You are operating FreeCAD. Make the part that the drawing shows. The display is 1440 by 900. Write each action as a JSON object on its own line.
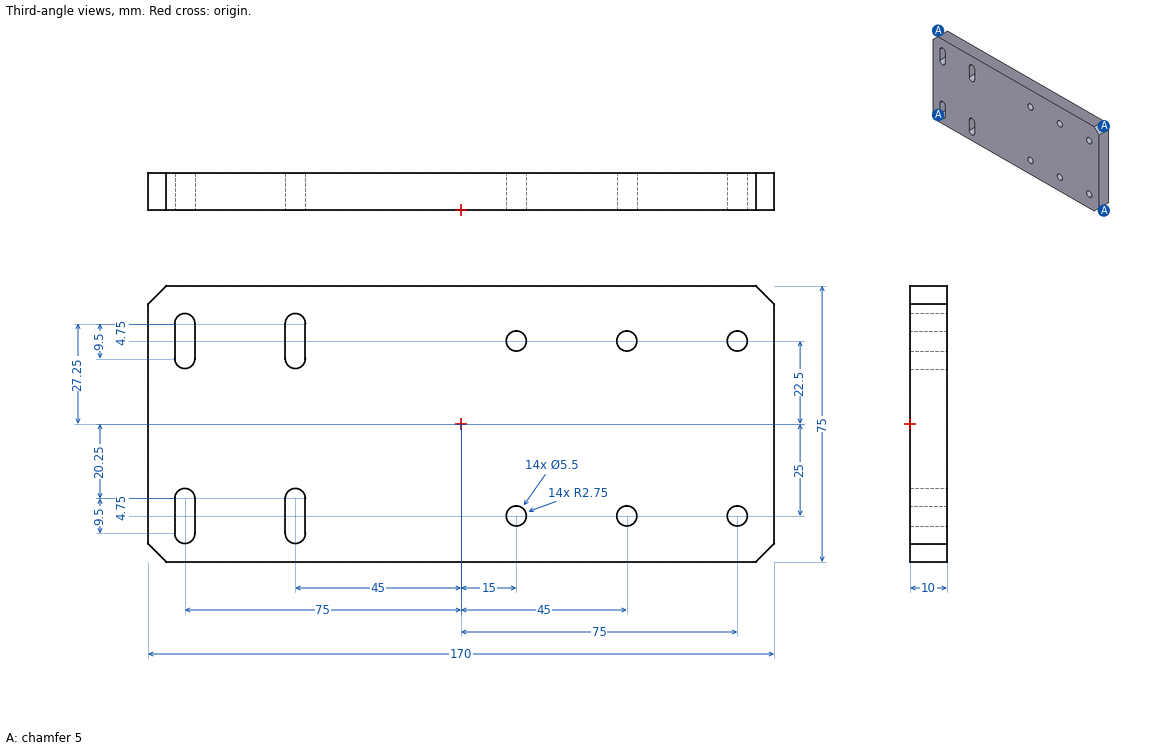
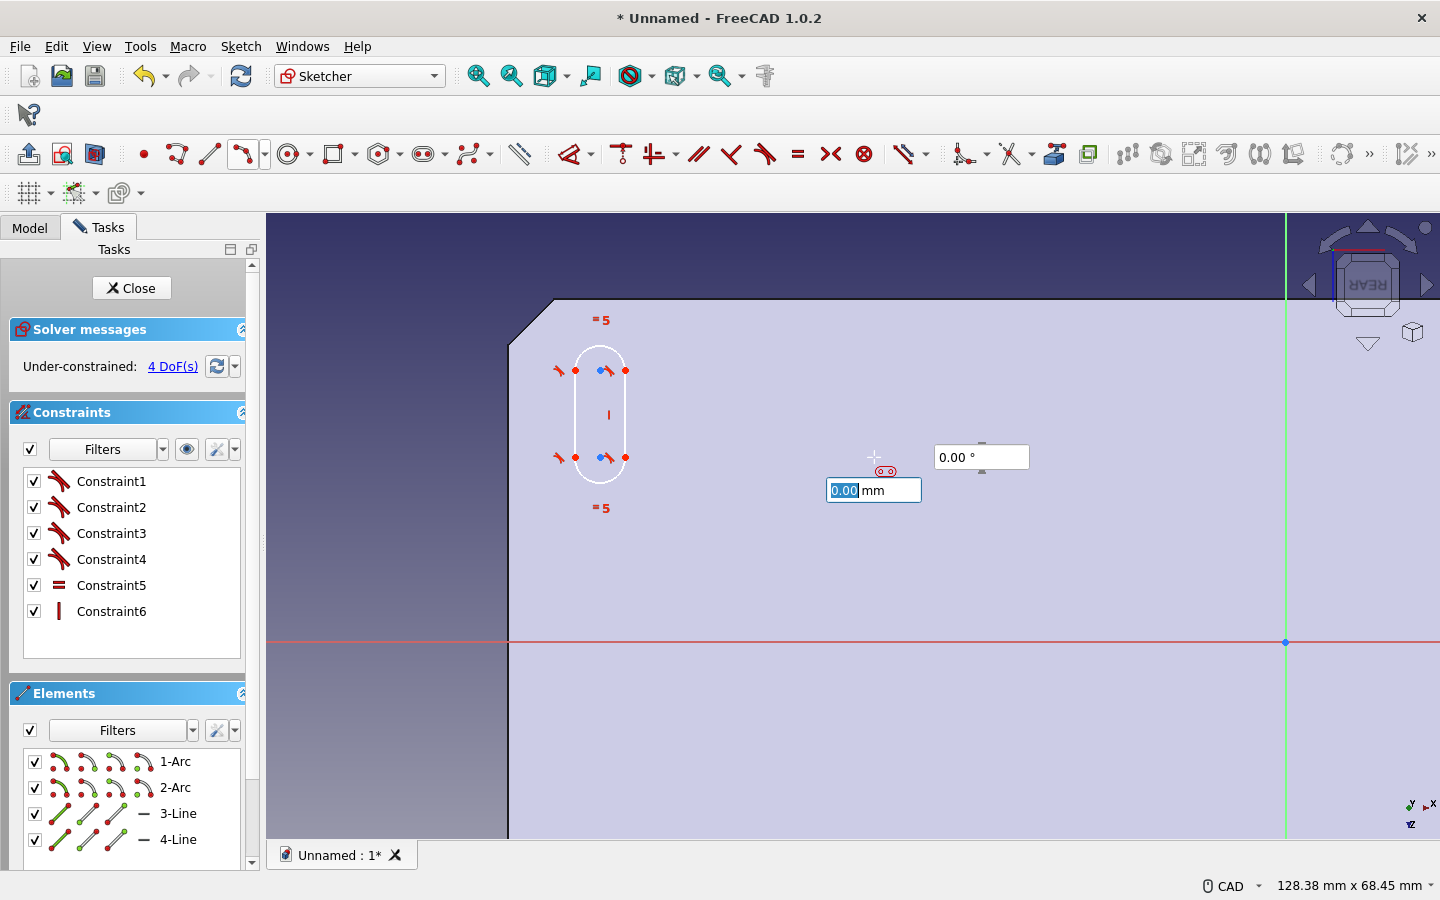
{"action": "left_click", "coordinate": [874, 370]}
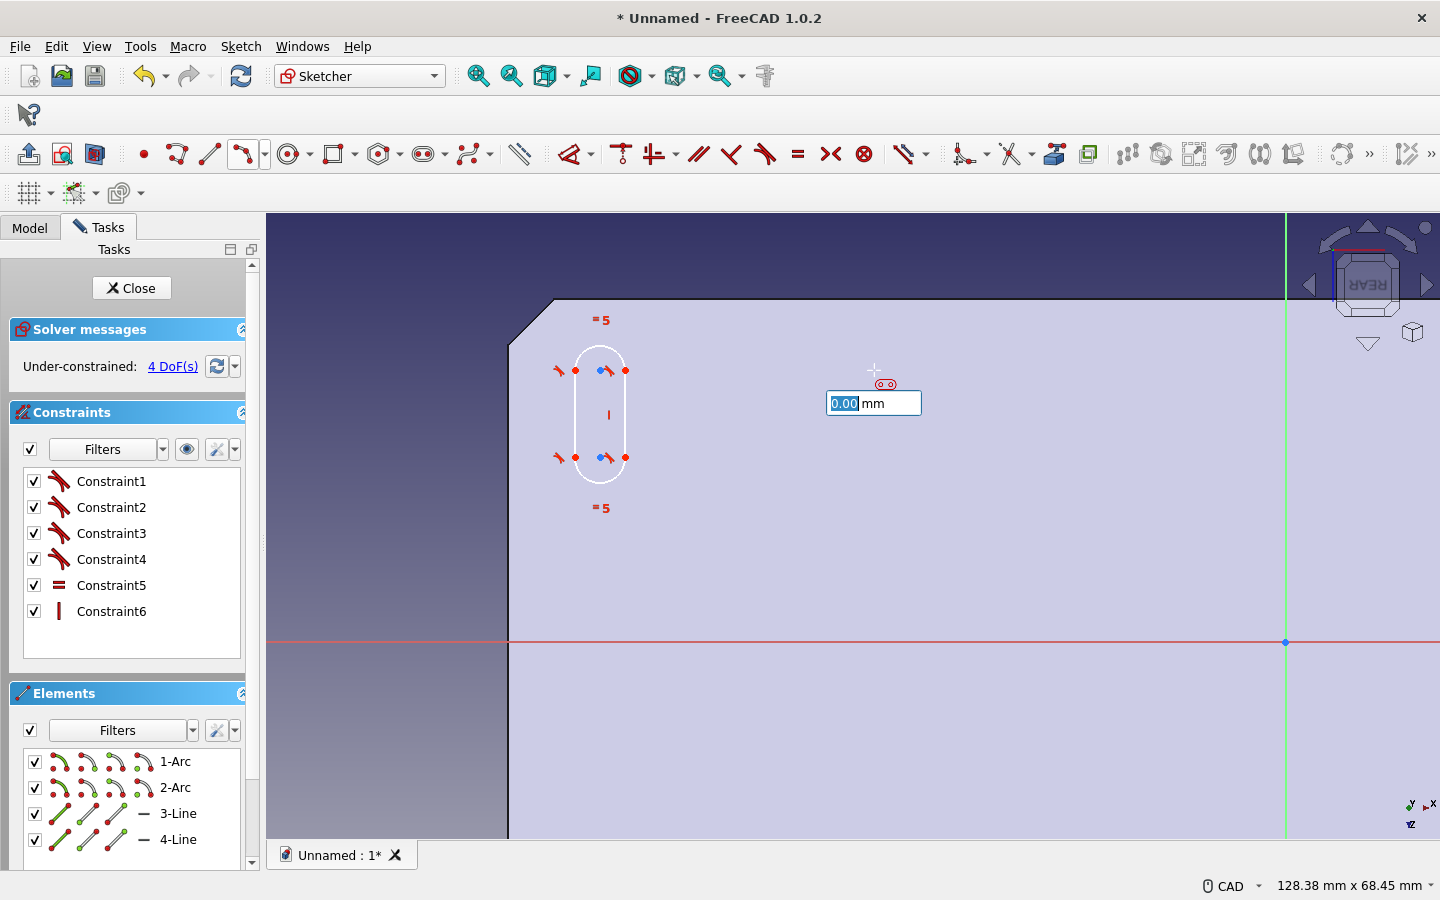
{"action": "left_click", "coordinate": [899, 414]}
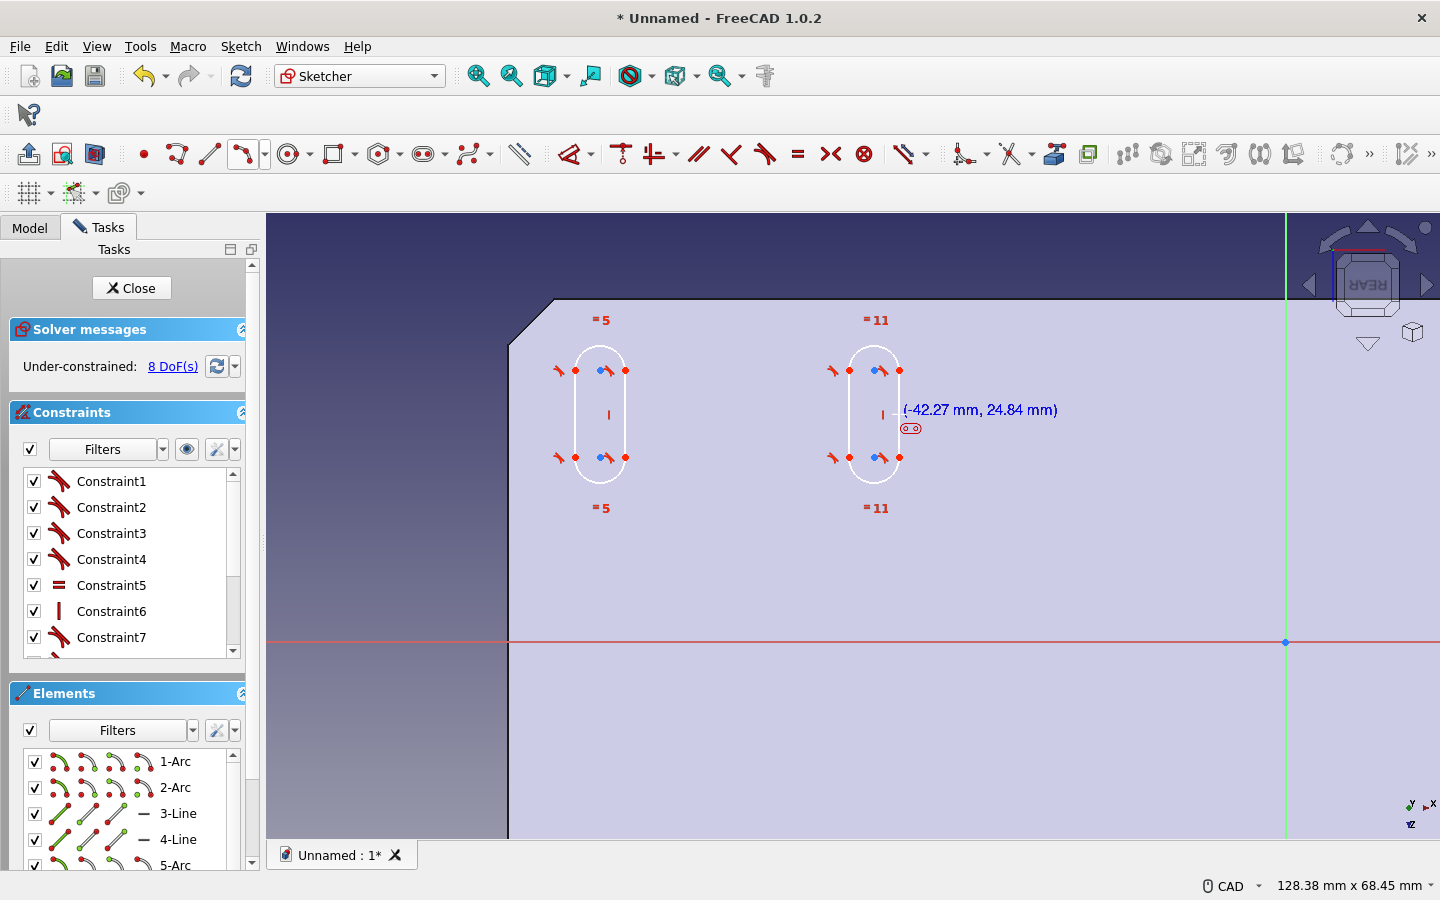
{"action": "scroll", "coordinate": [376, 441], "scroll_direction": "down", "scroll_amount": 4}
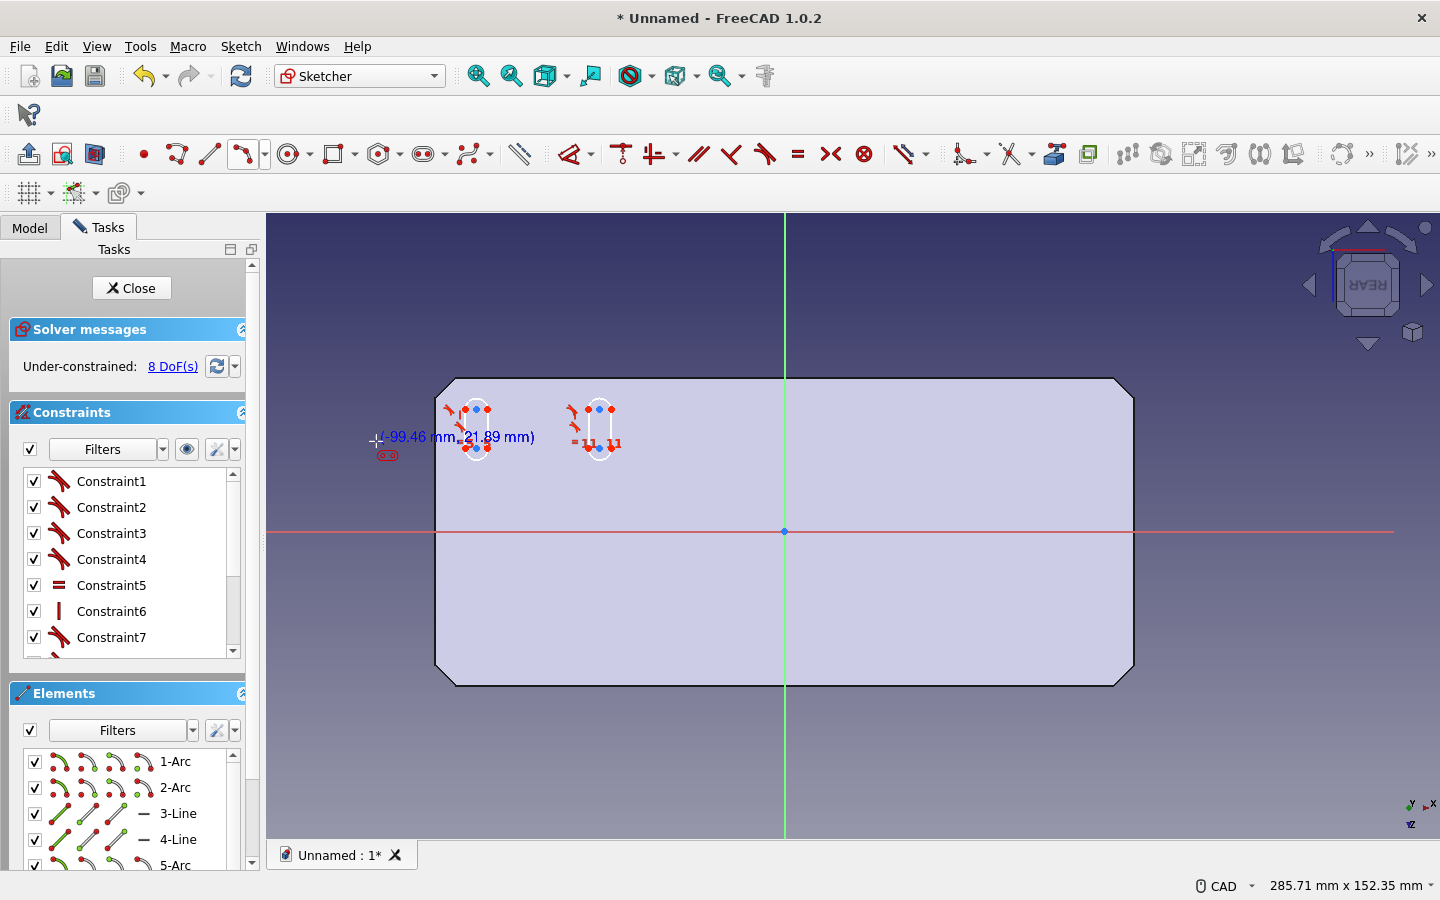
{"action": "scroll", "coordinate": [477, 644], "scroll_direction": "up", "scroll_amount": 4}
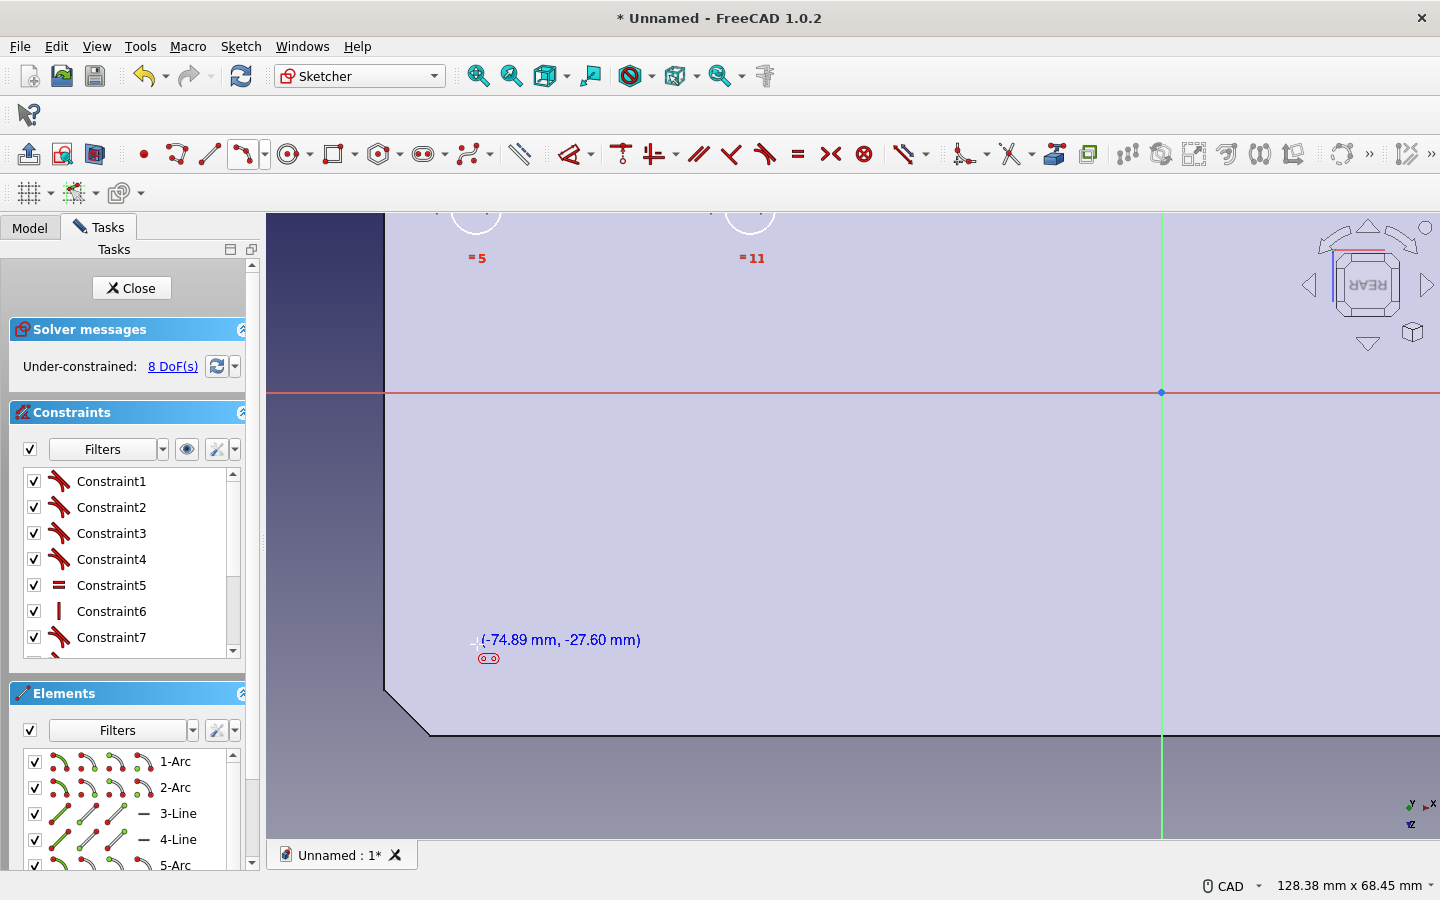
{"action": "left_click", "coordinate": [476, 642]}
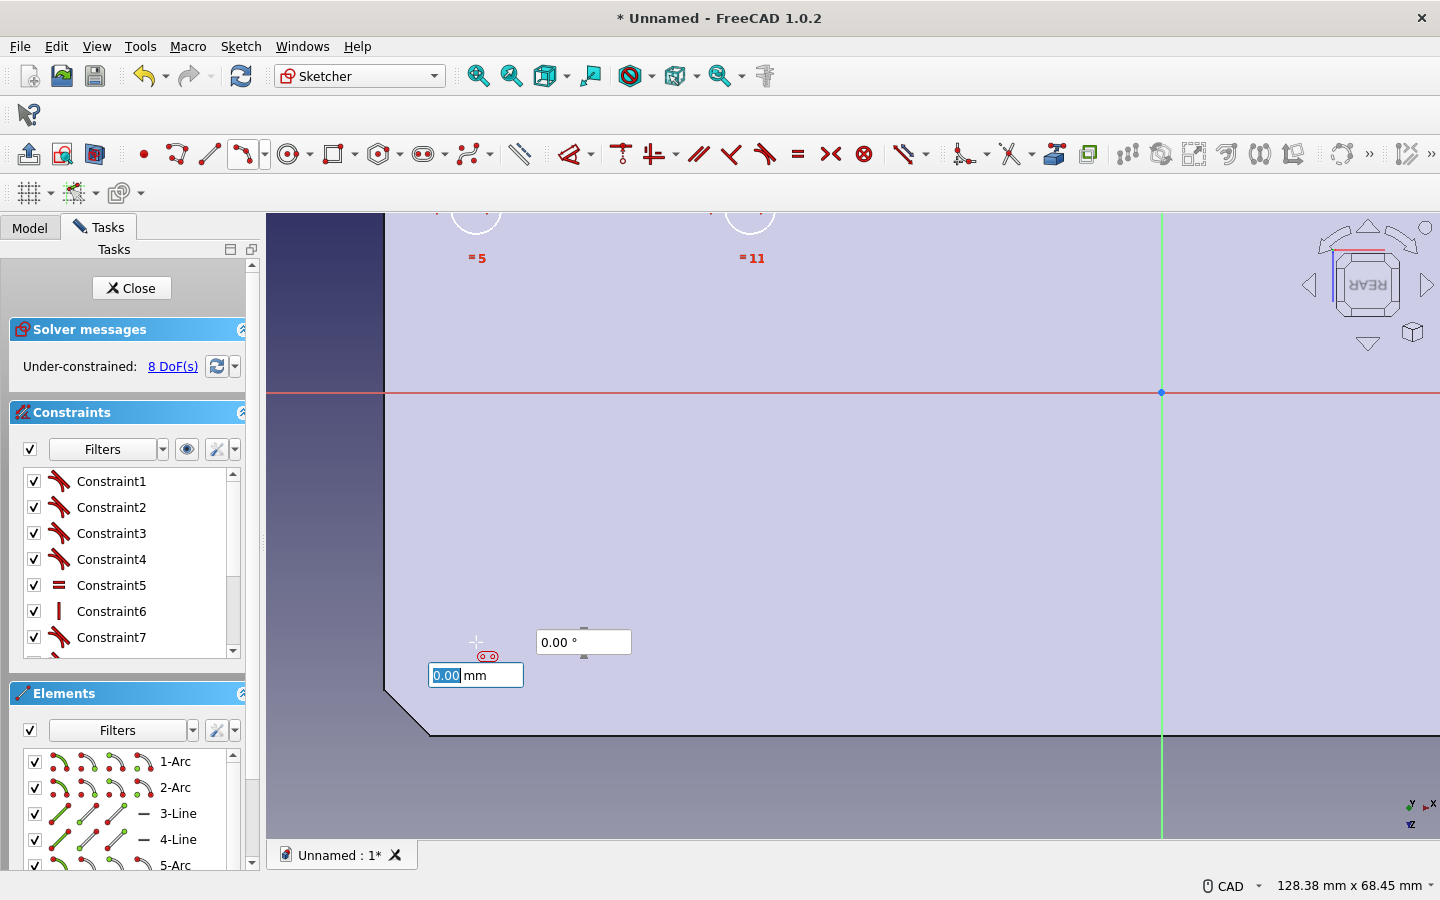
{"action": "left_click", "coordinate": [476, 555]}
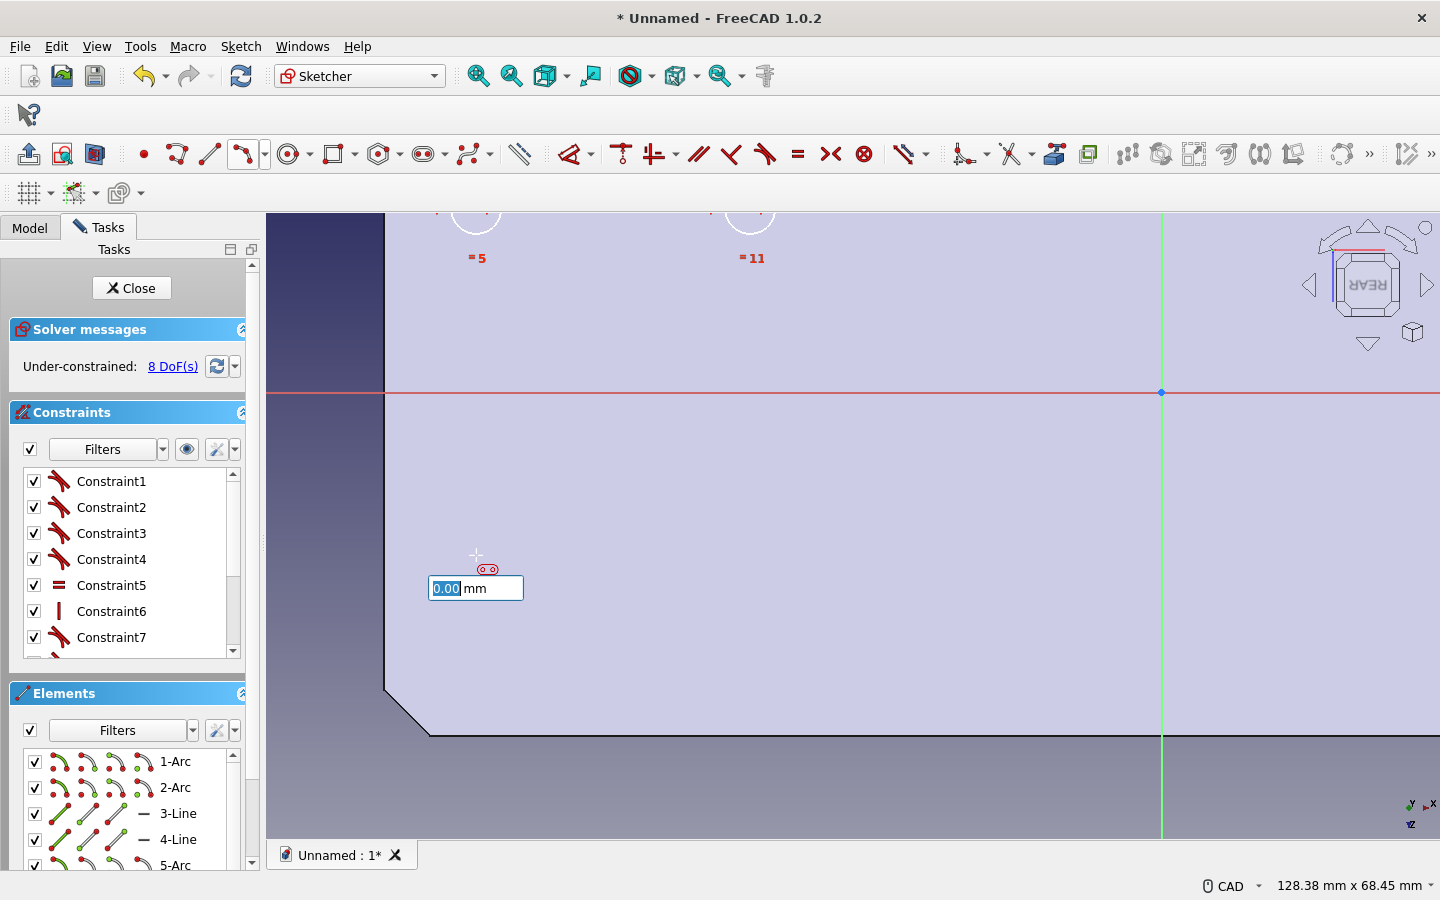
{"action": "left_click", "coordinate": [501, 599]}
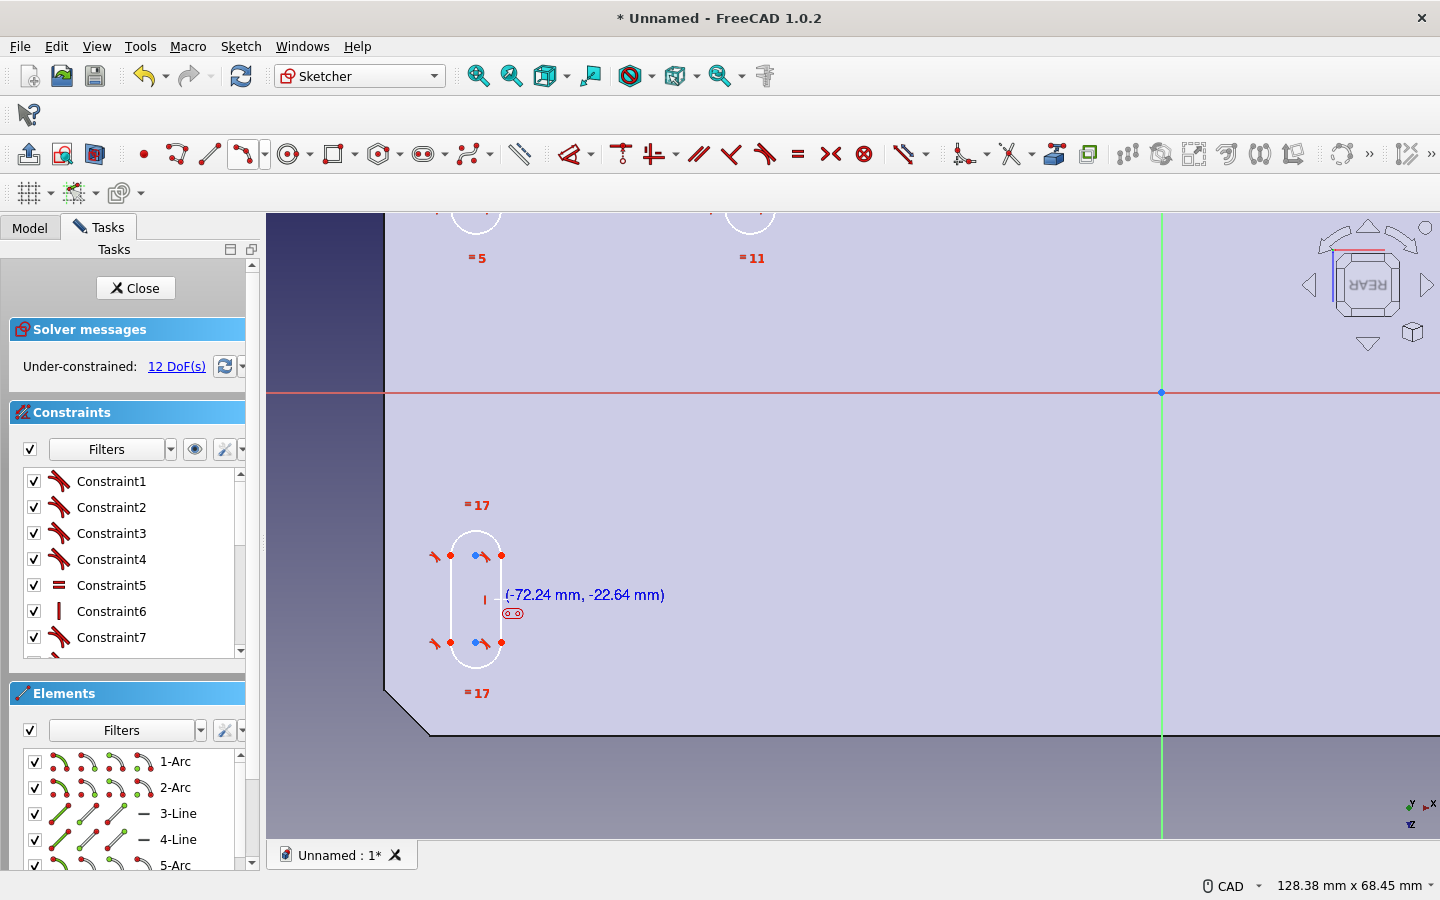
{"action": "left_click", "coordinate": [750, 642]}